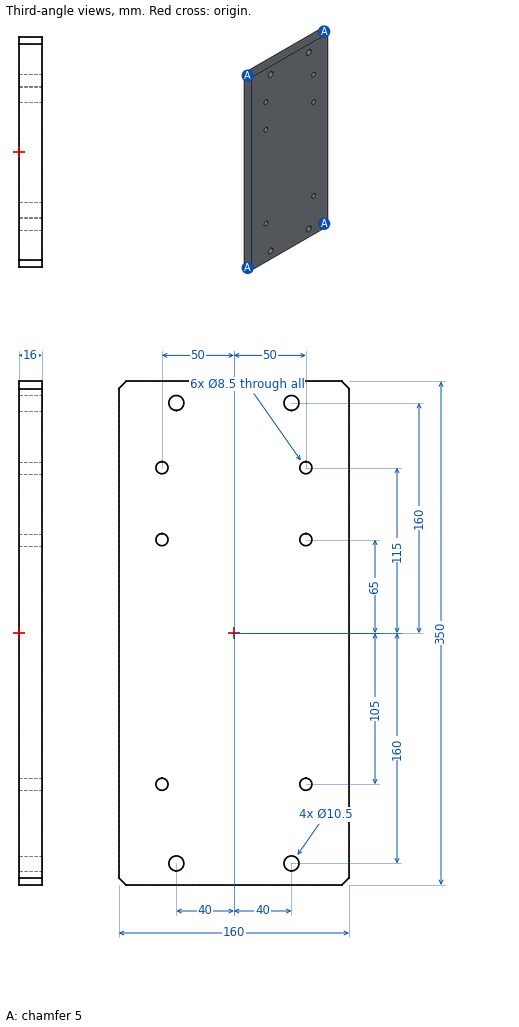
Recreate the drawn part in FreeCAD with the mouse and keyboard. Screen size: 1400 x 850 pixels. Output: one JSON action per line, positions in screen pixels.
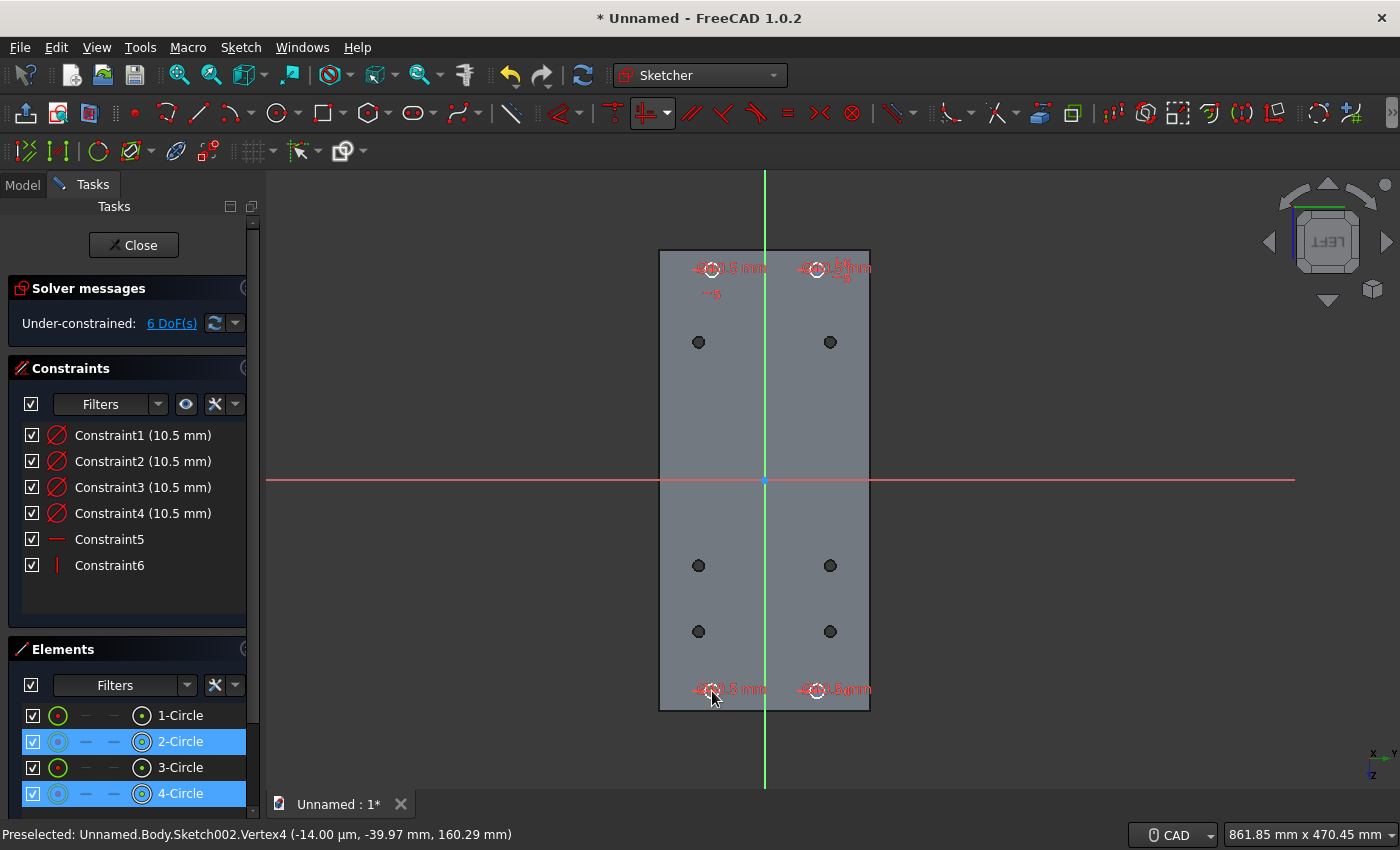
{"action": "key", "text": "v"}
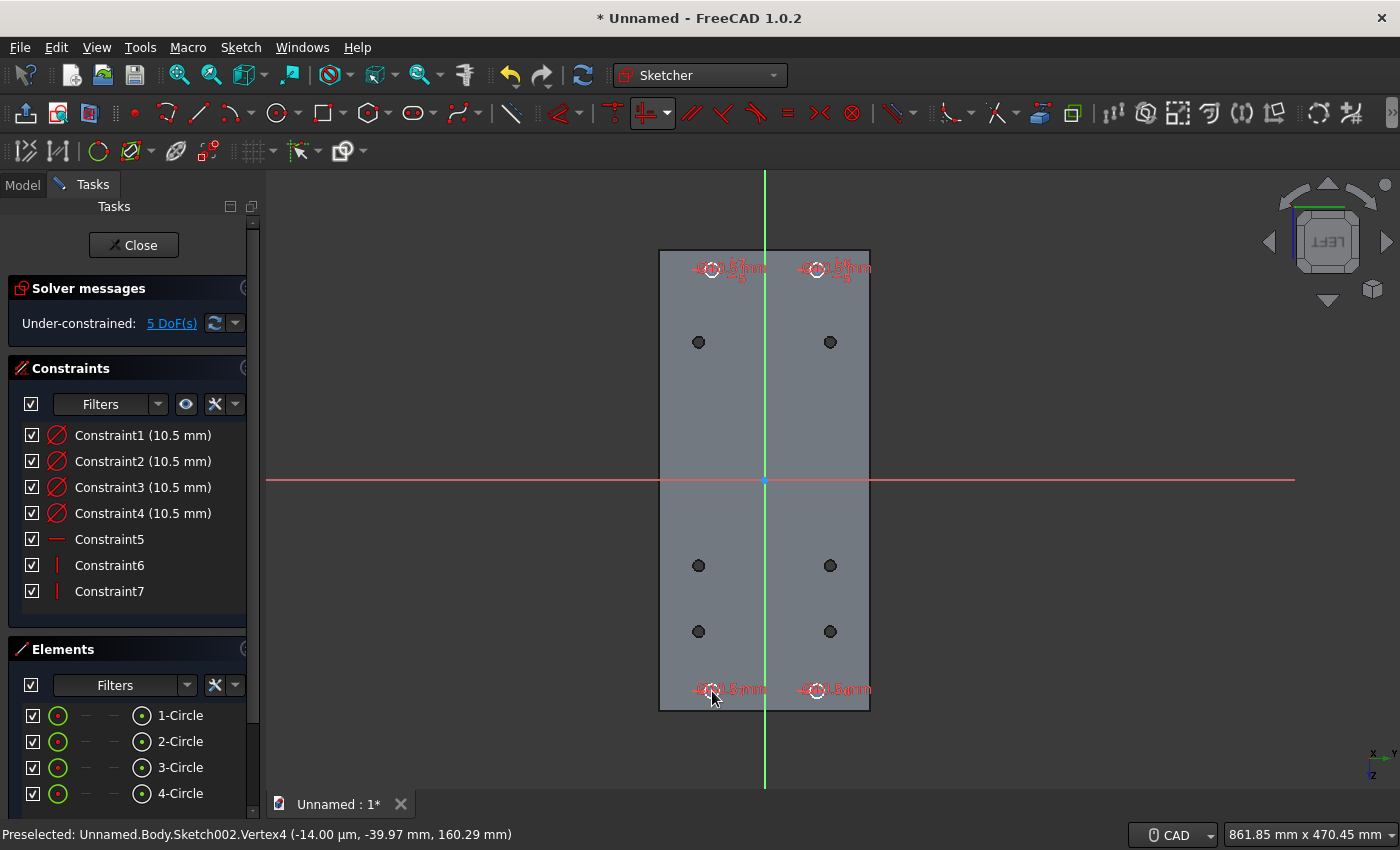
{"action": "left_click", "coordinate": [817, 691]}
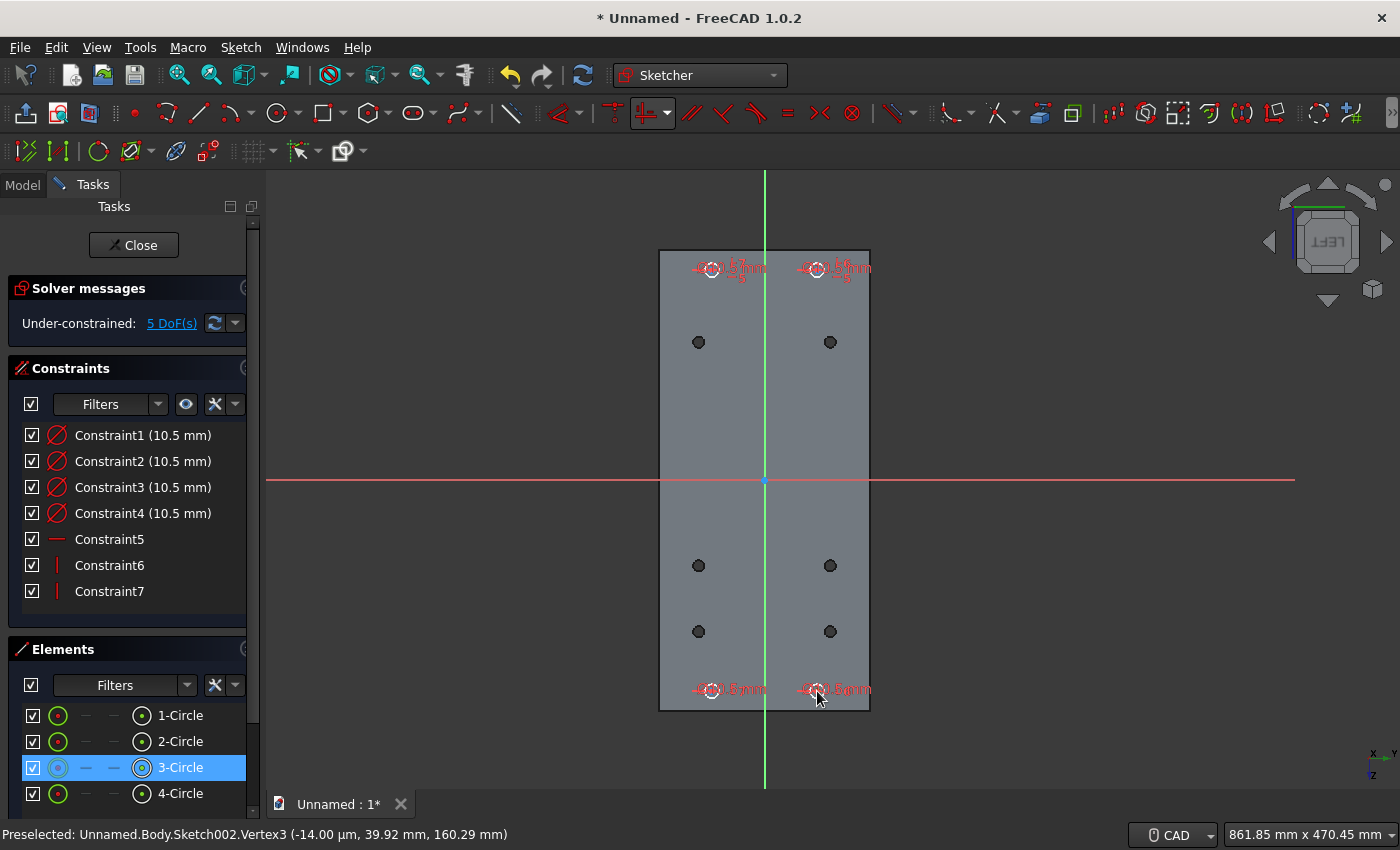
{"action": "left_click", "coordinate": [712, 691]}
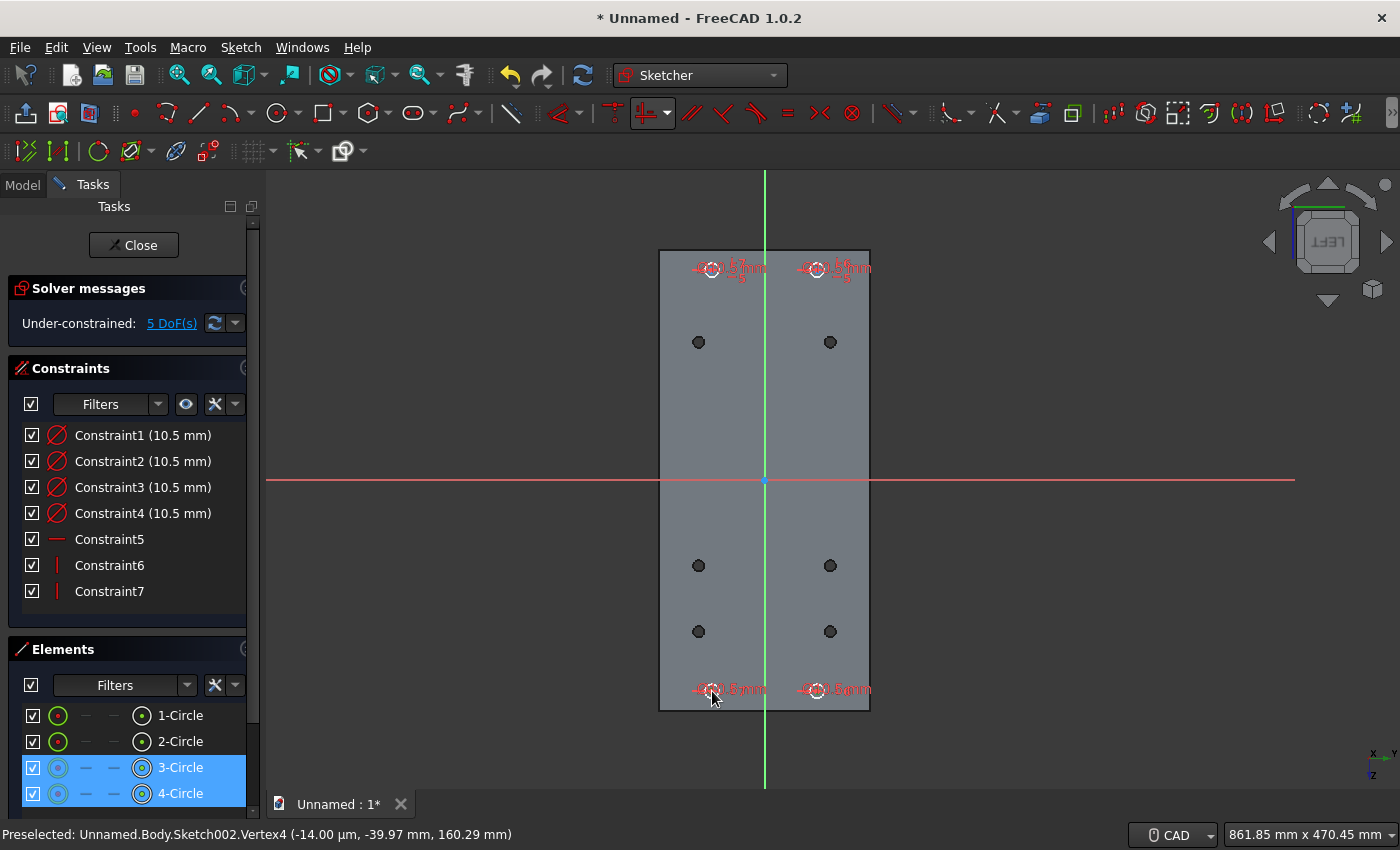
{"action": "left_click", "coordinate": [670, 114]}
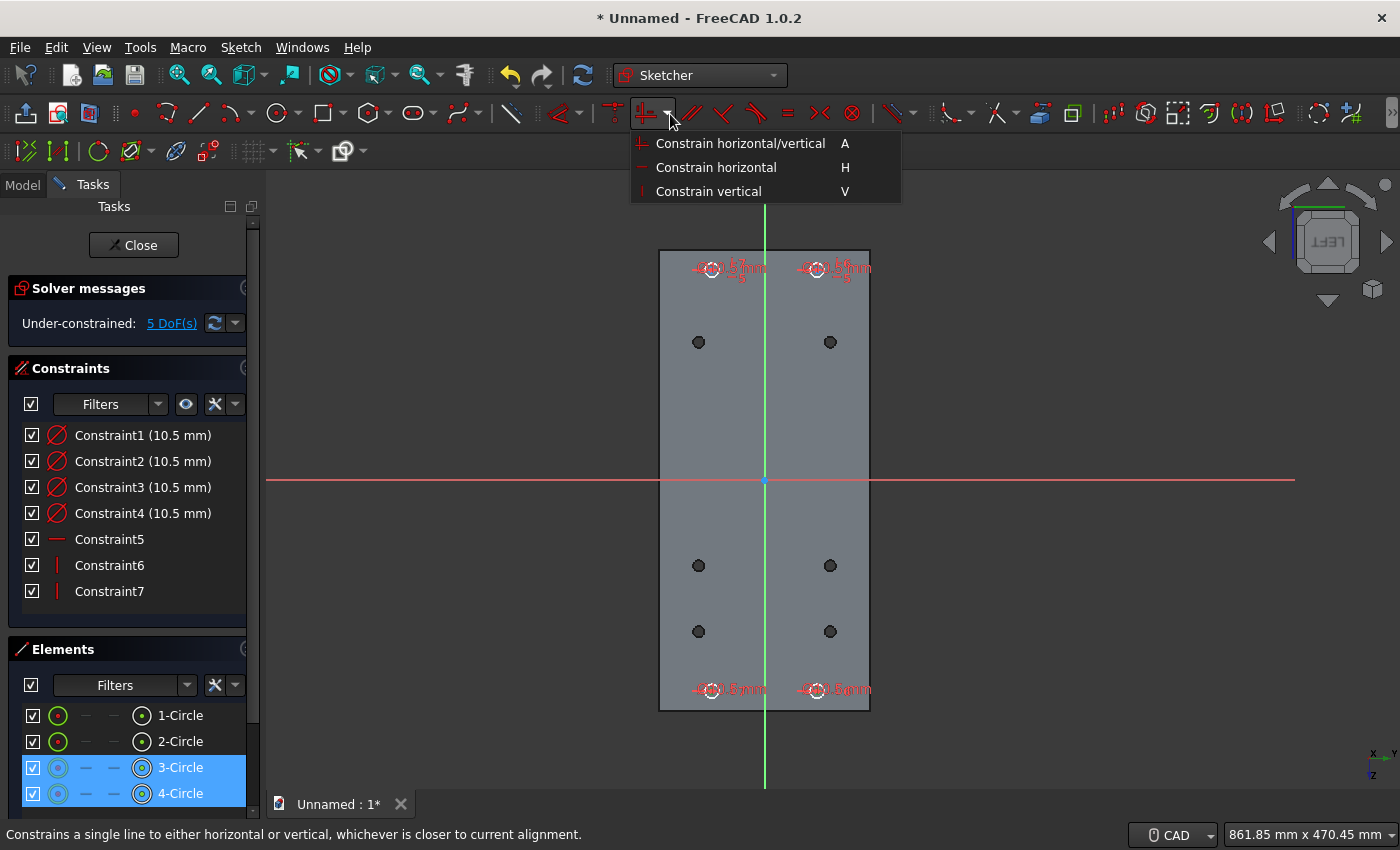
{"action": "left_click", "coordinate": [766, 167]}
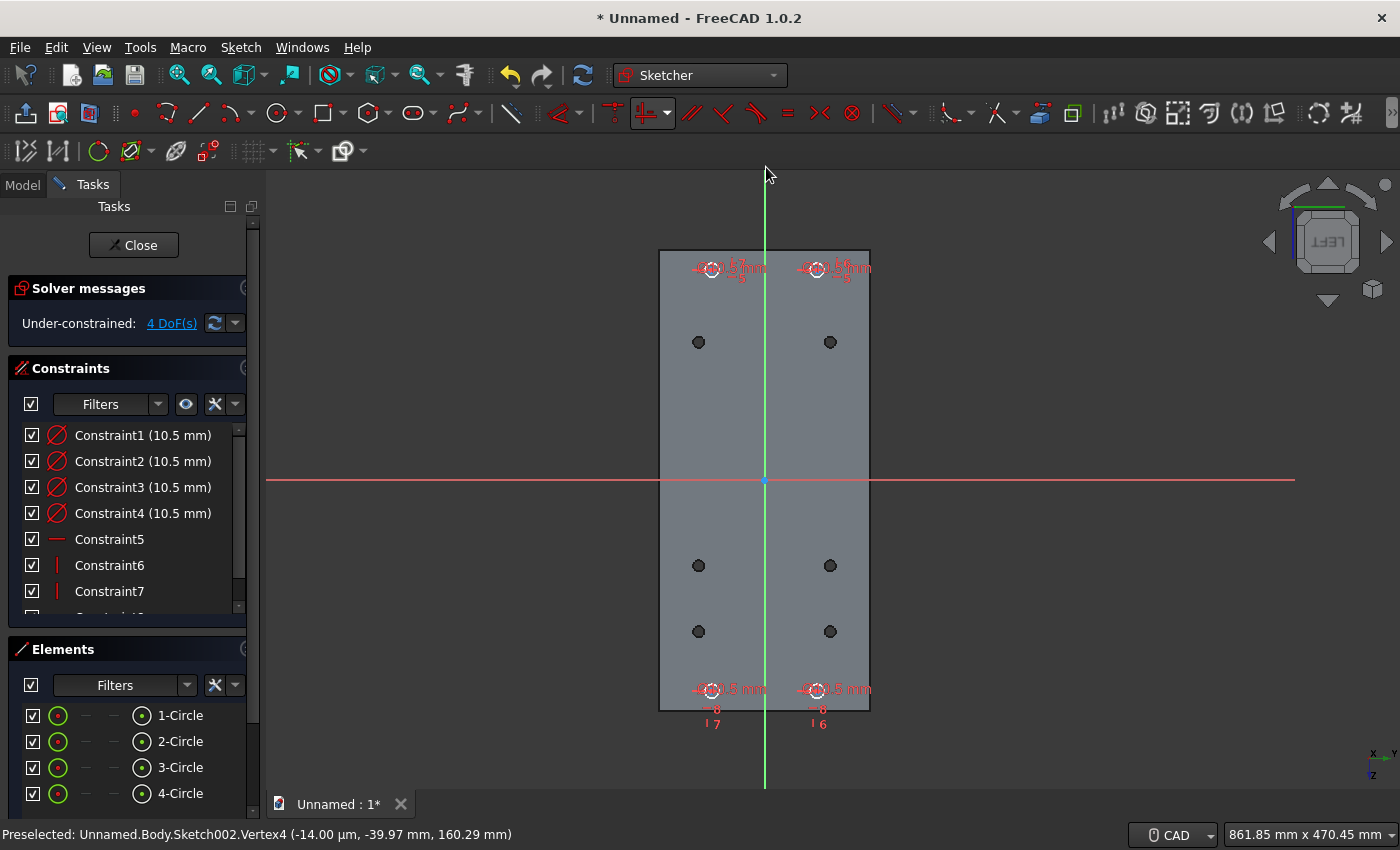
{"action": "left_click", "coordinate": [558, 114]}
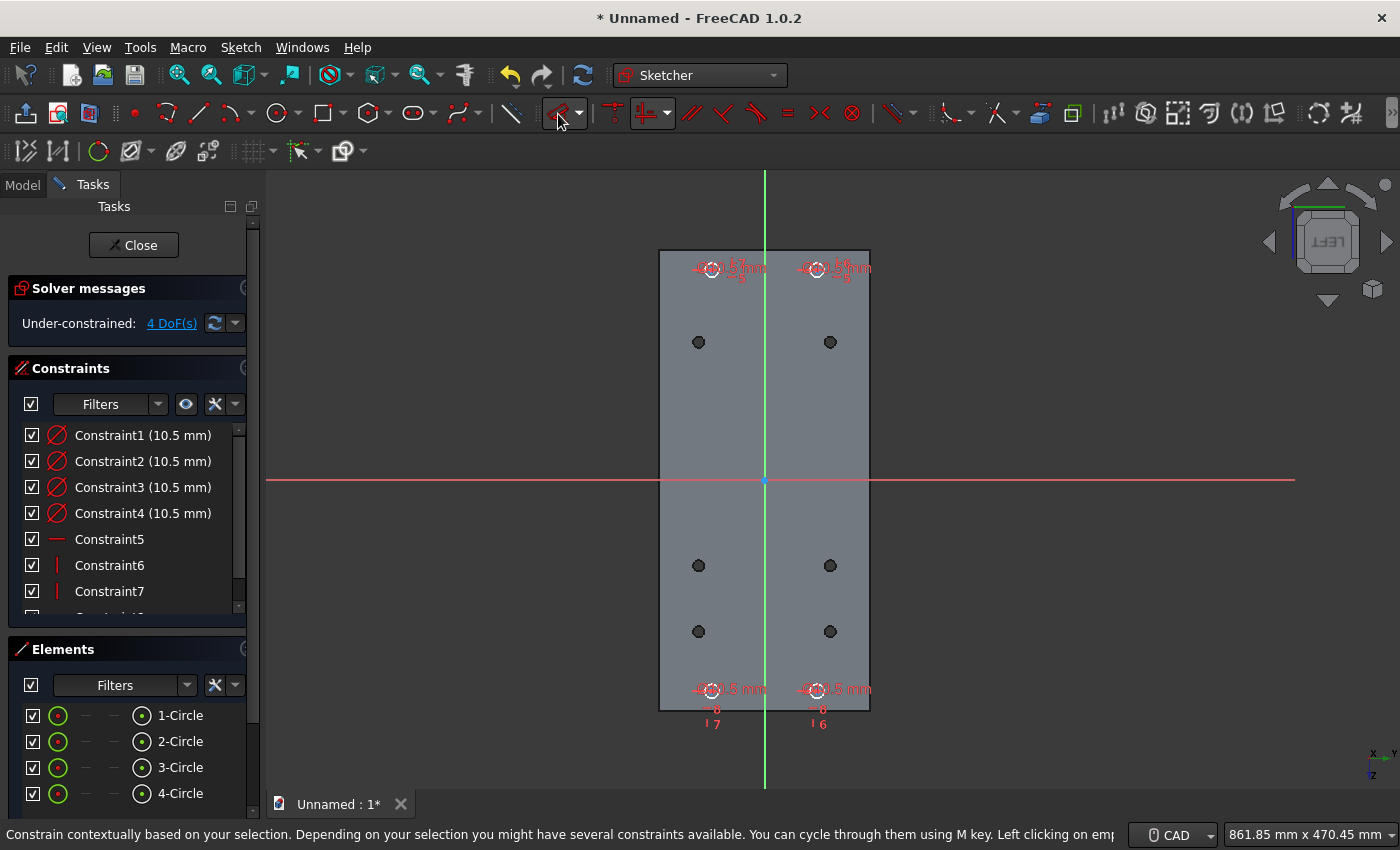
{"action": "left_click", "coordinate": [817, 270]}
{"action": "left_click", "coordinate": [791, 236]}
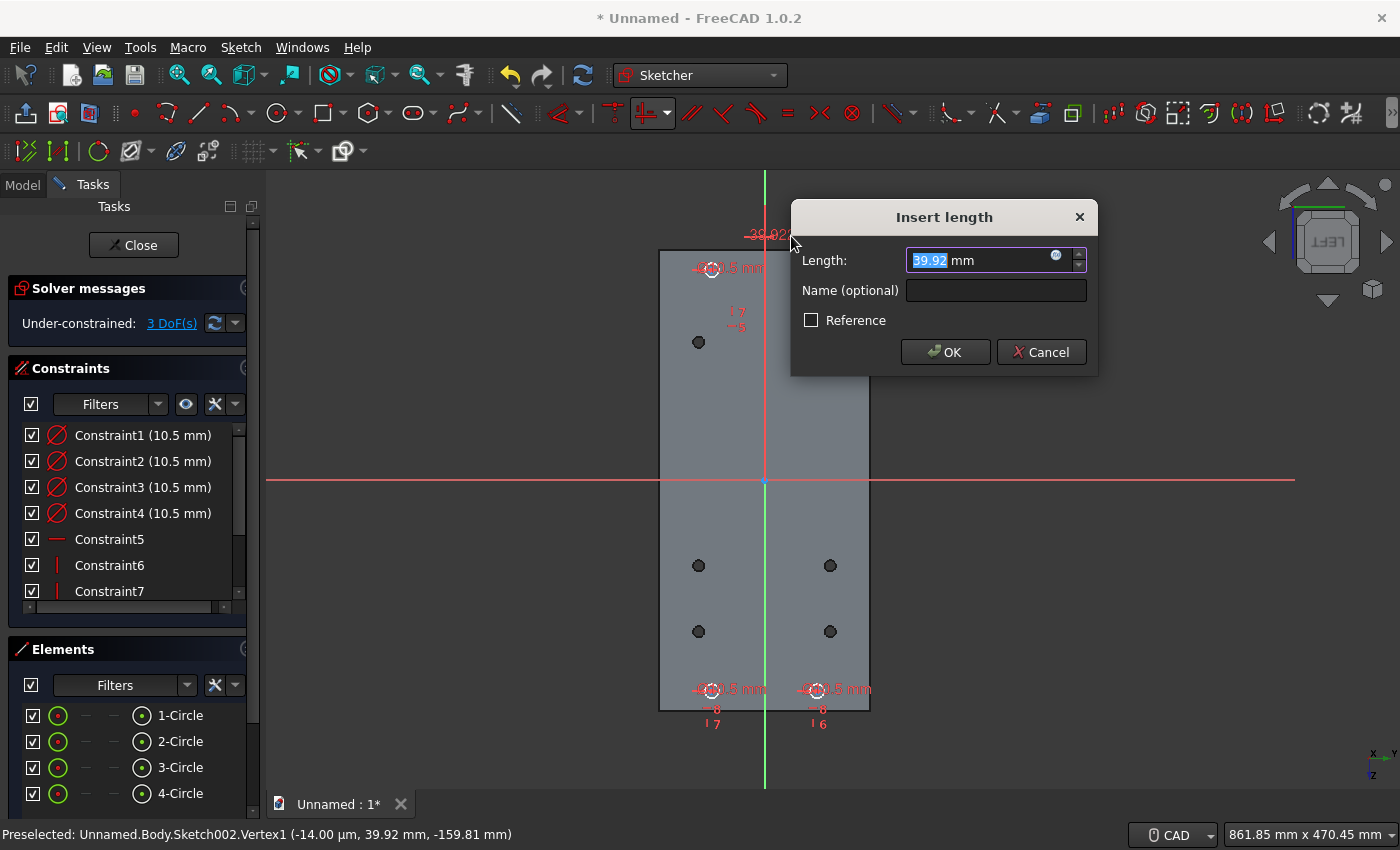
{"action": "type", "text": "40"}
{"action": "key", "text": "Return"}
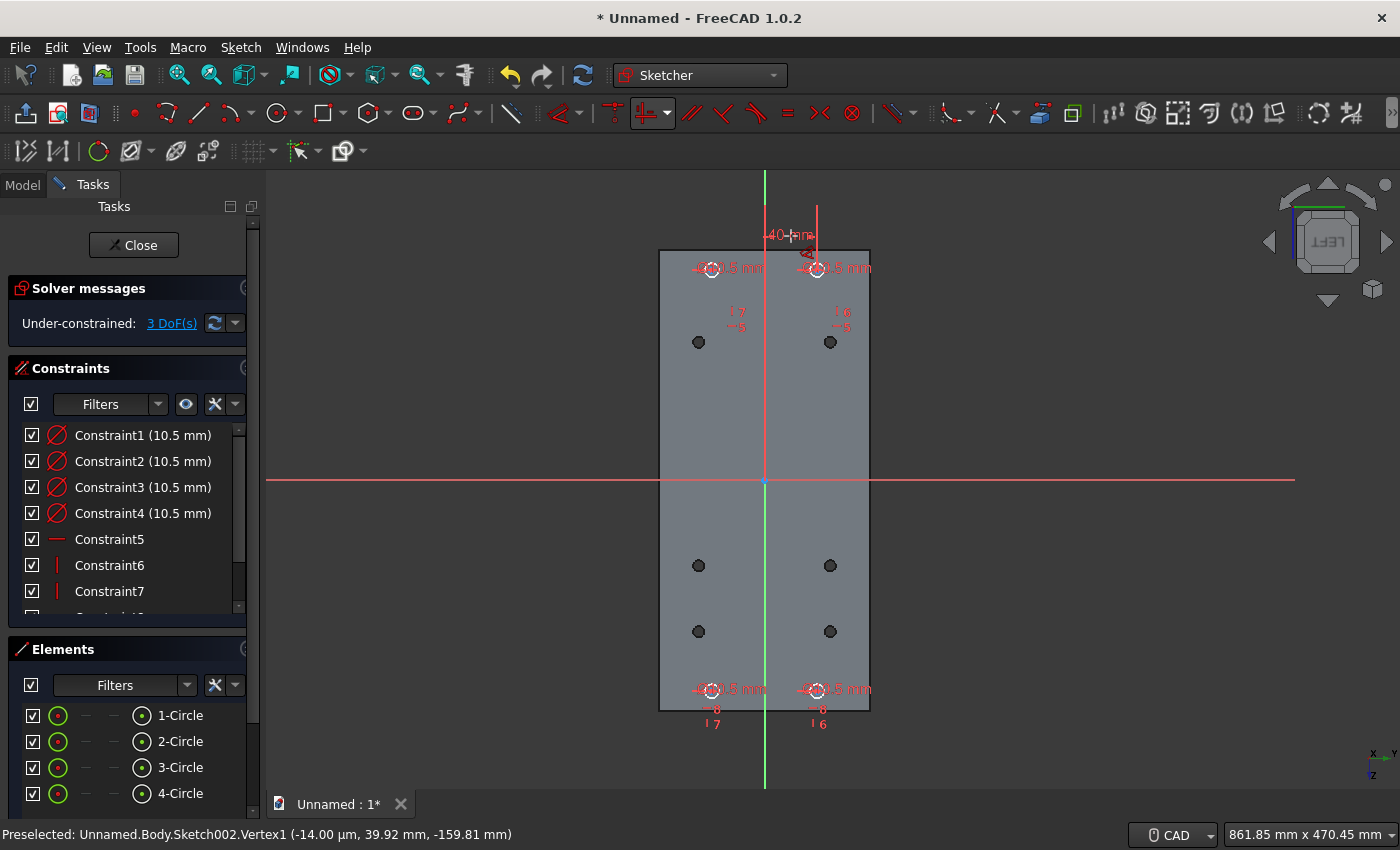
{"action": "left_click", "coordinate": [712, 270]}
{"action": "left_click", "coordinate": [720, 236]}